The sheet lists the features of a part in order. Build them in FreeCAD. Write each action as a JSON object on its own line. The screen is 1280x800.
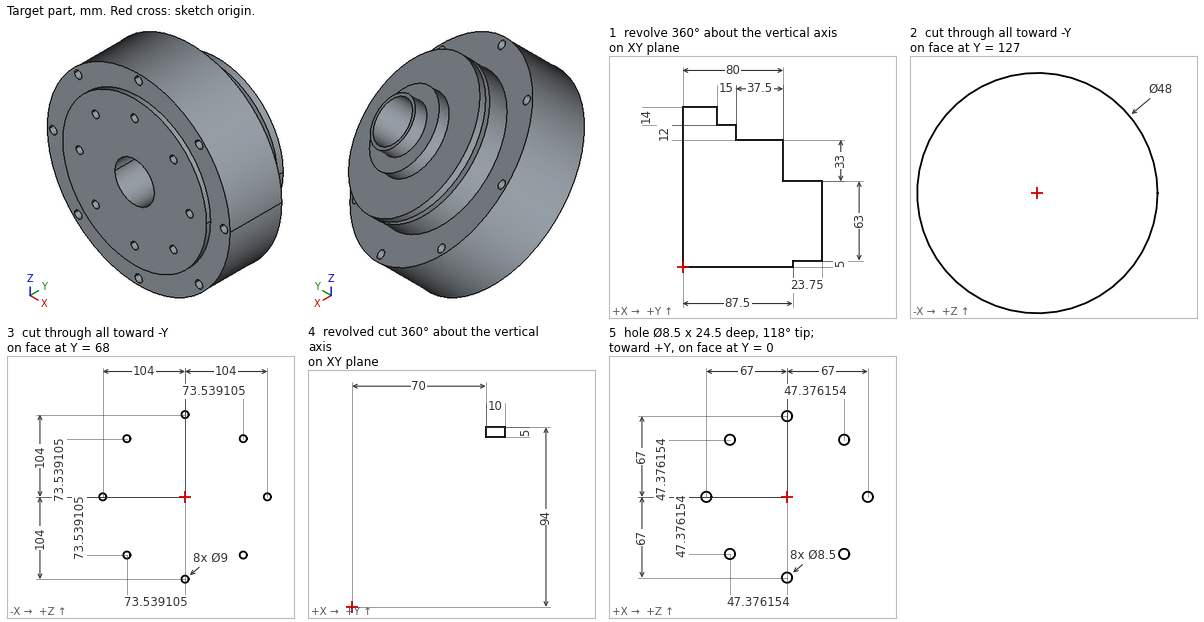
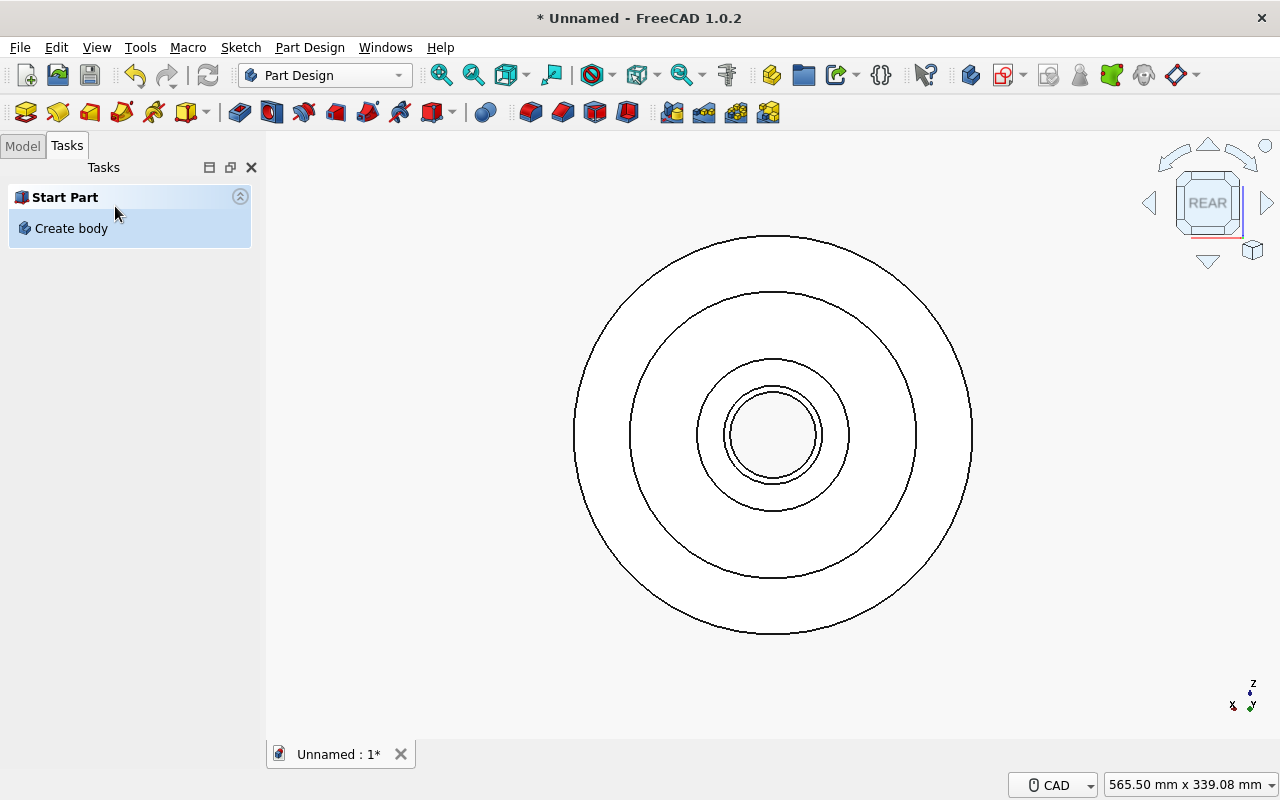
{"action": "left_click", "coordinate": [602, 434]}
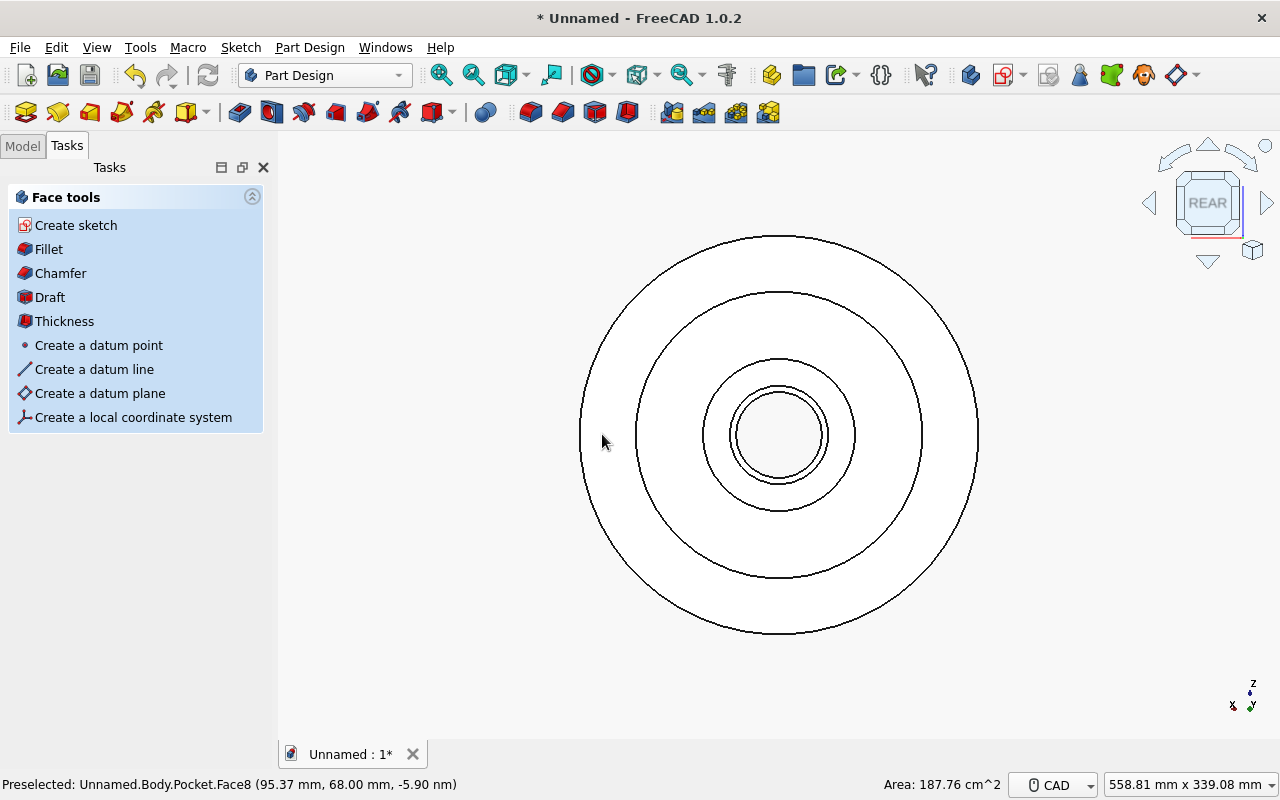
{"action": "left_click", "coordinate": [1004, 76]}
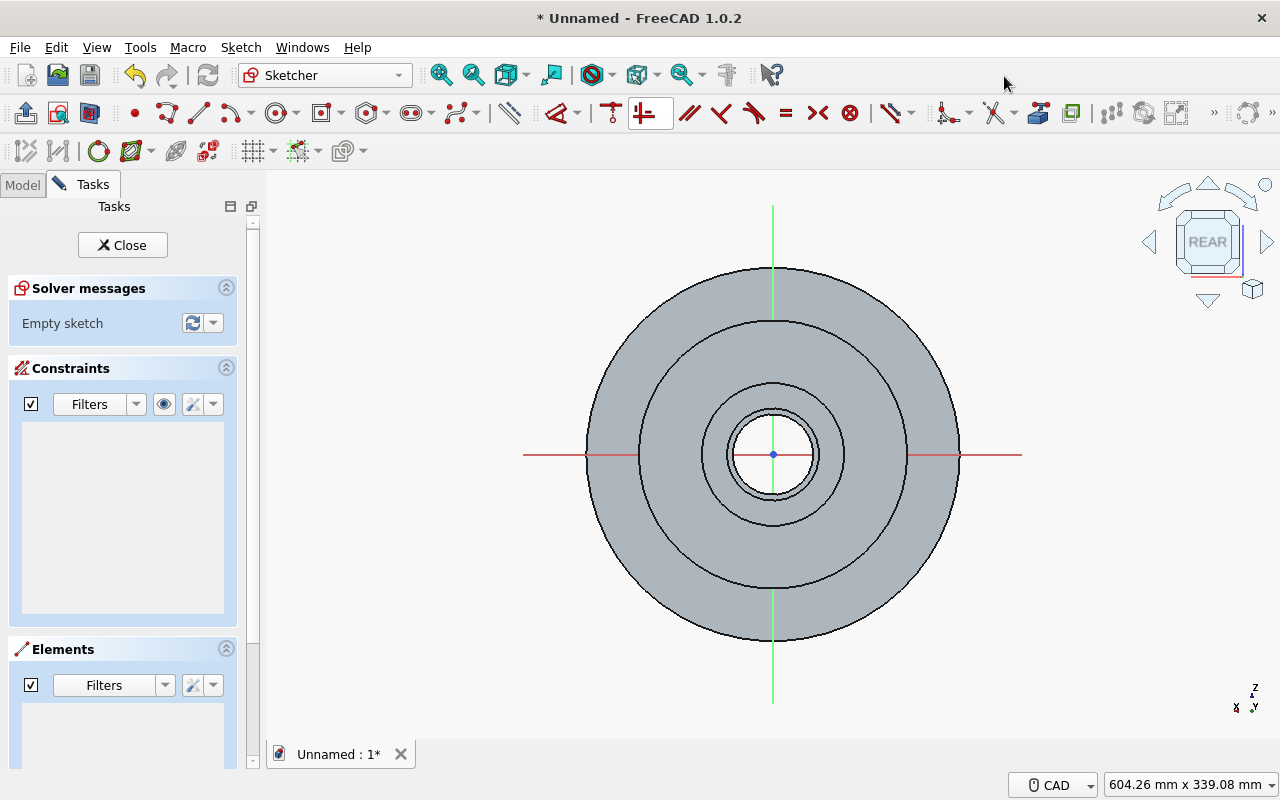
{"action": "left_click", "coordinate": [276, 114]}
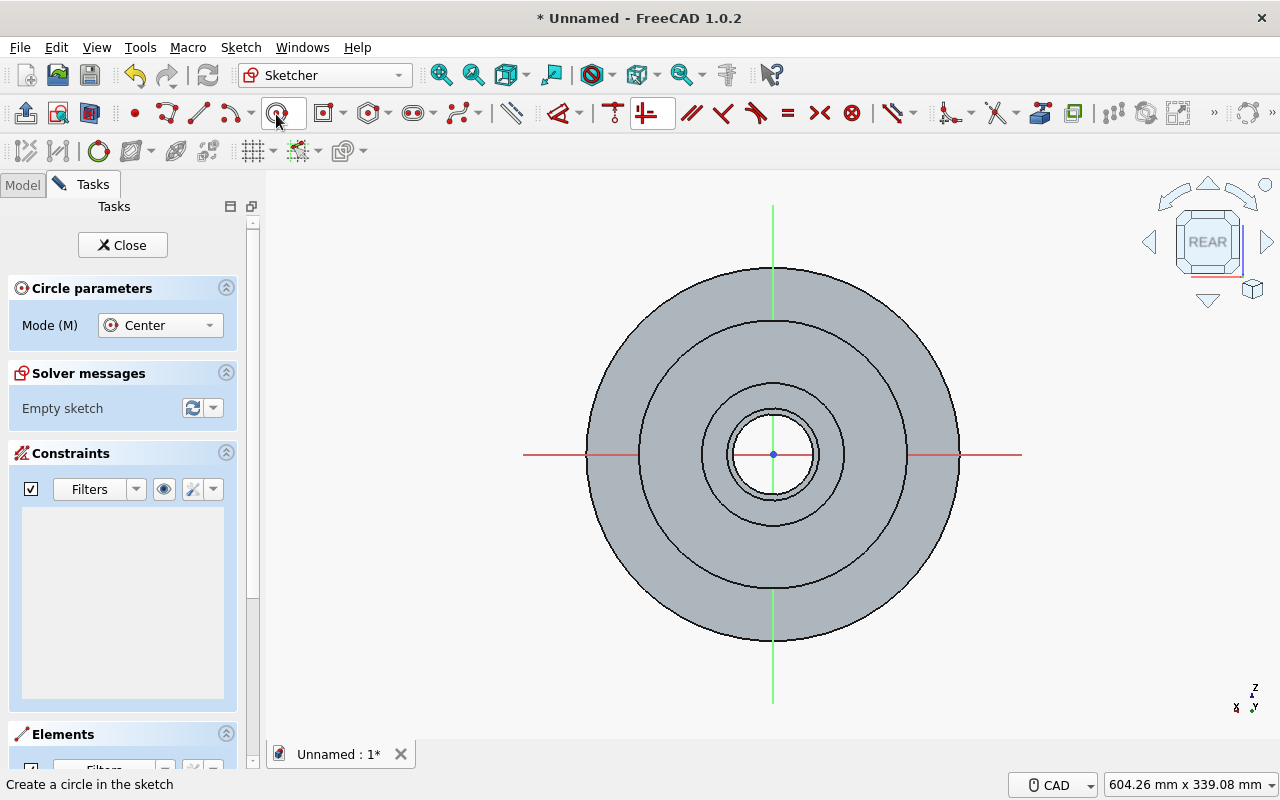
{"action": "scroll", "coordinate": [773, 629], "scroll_direction": "up", "scroll_amount": 6}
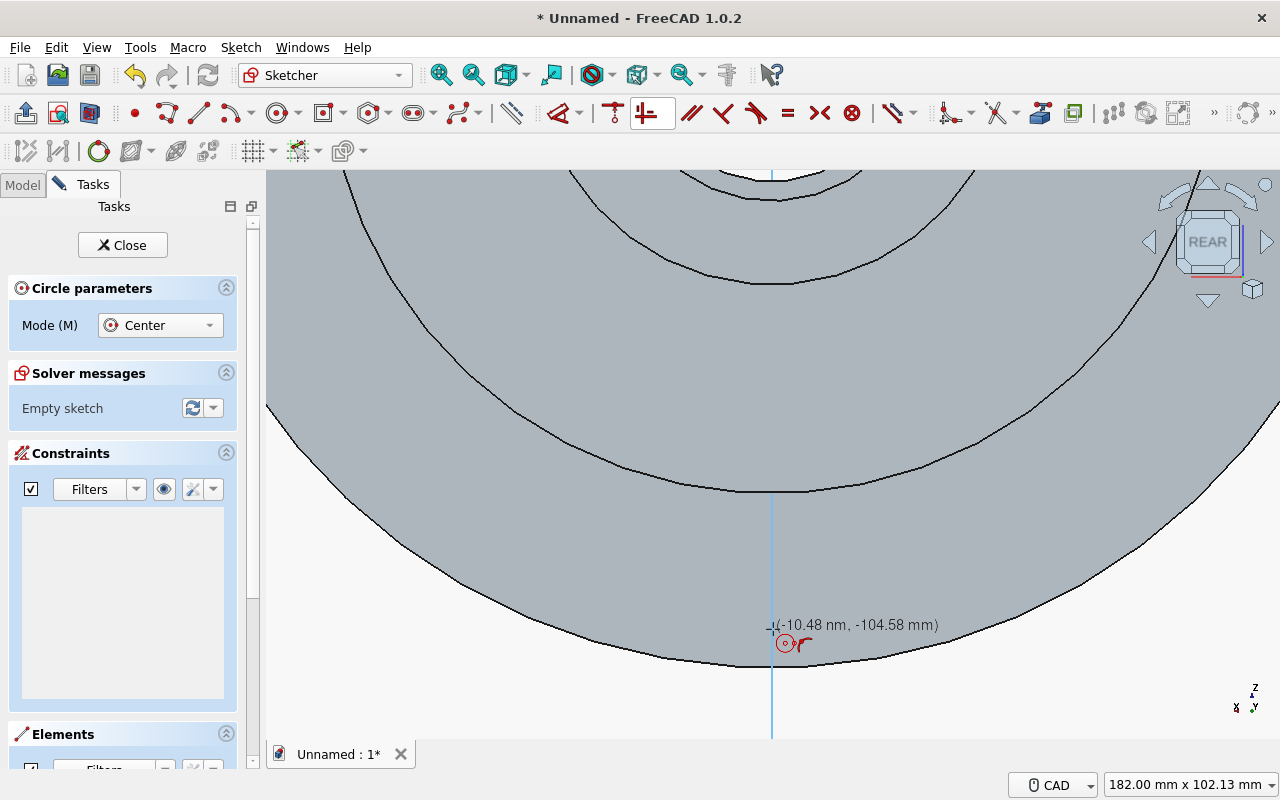
{"action": "left_click", "coordinate": [772, 627]}
{"action": "left_click", "coordinate": [790, 609]}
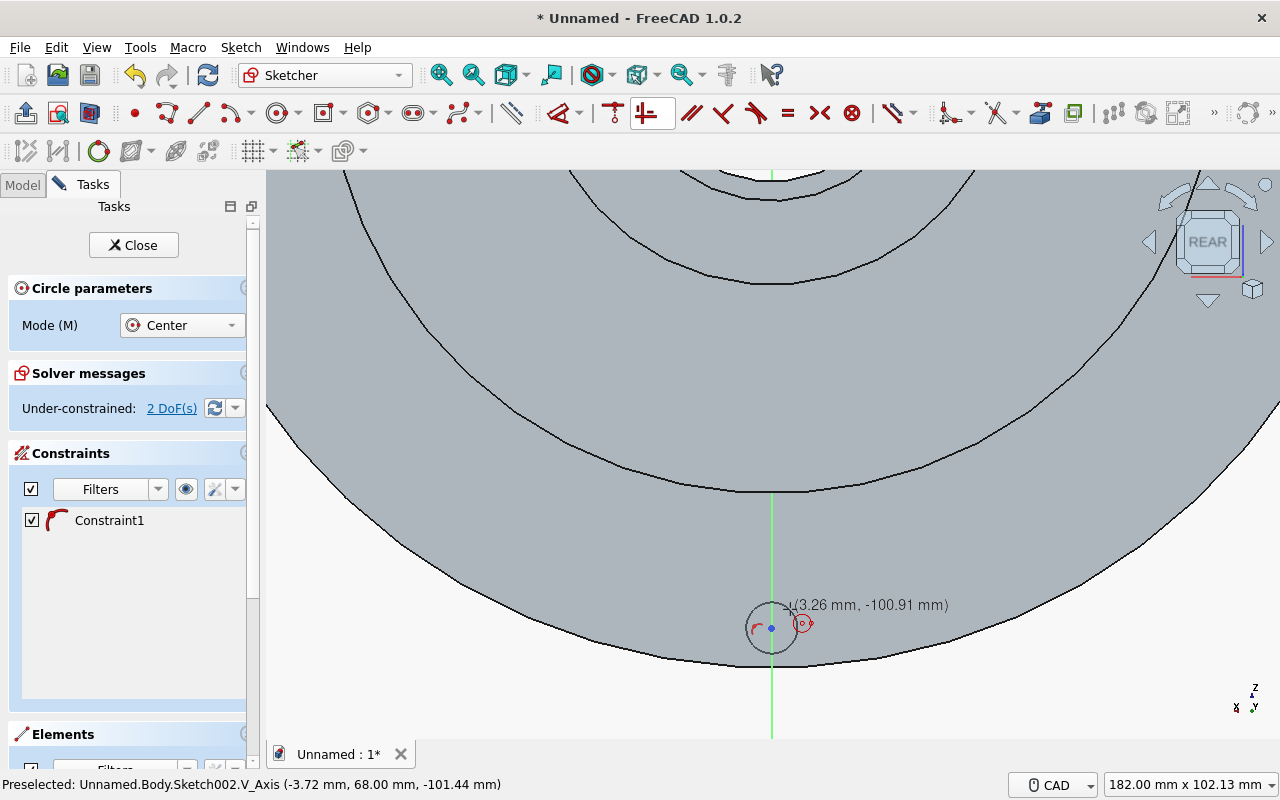
{"action": "left_click", "coordinate": [362, 457]}
{"action": "left_click", "coordinate": [380, 440]}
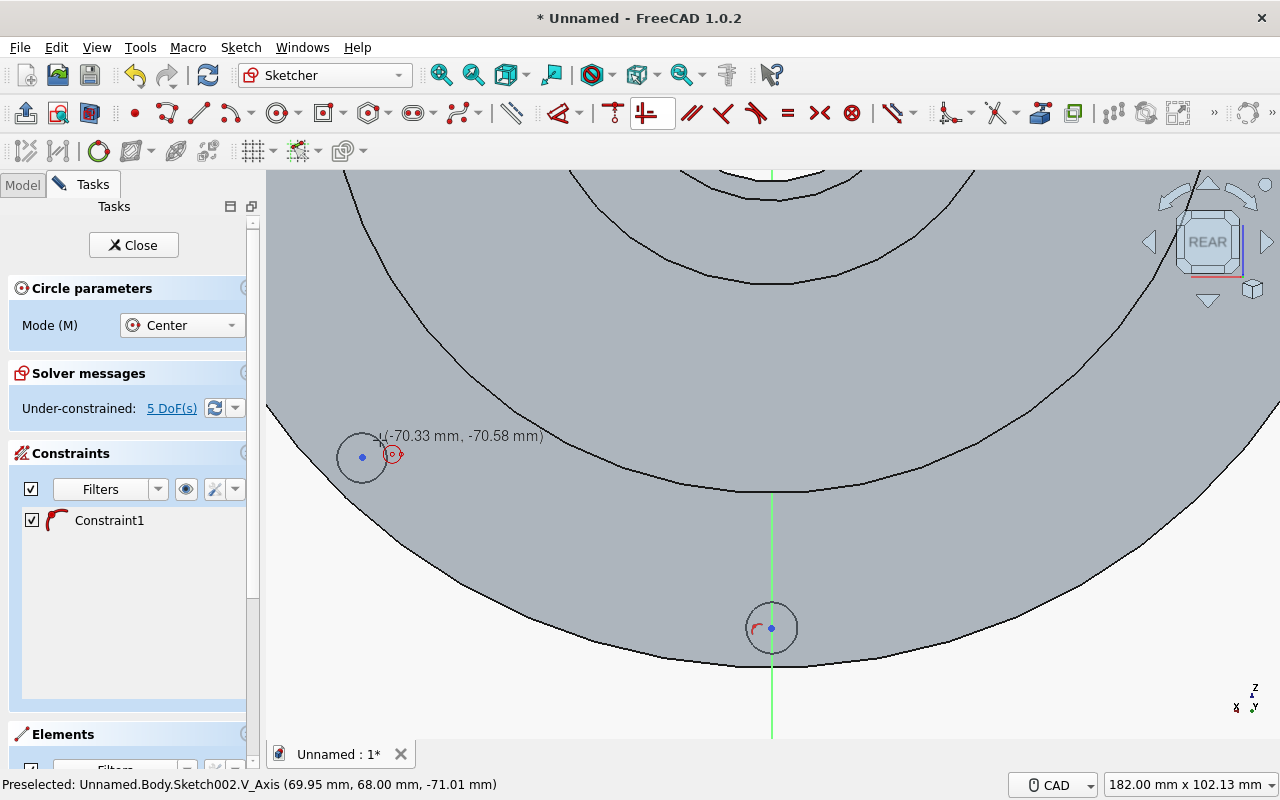
{"action": "scroll", "coordinate": [675, 630], "scroll_direction": "down", "scroll_amount": 6}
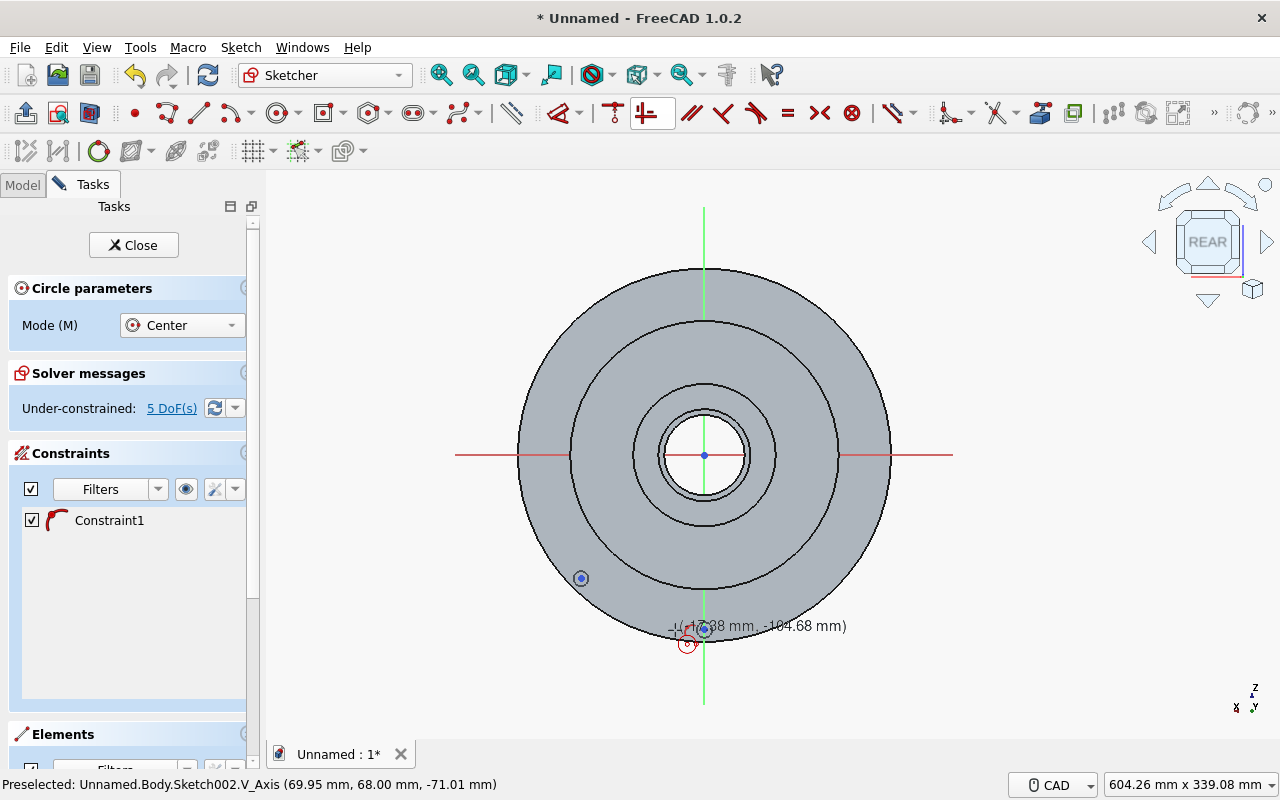
{"action": "scroll", "coordinate": [530, 455], "scroll_direction": "up", "scroll_amount": 6}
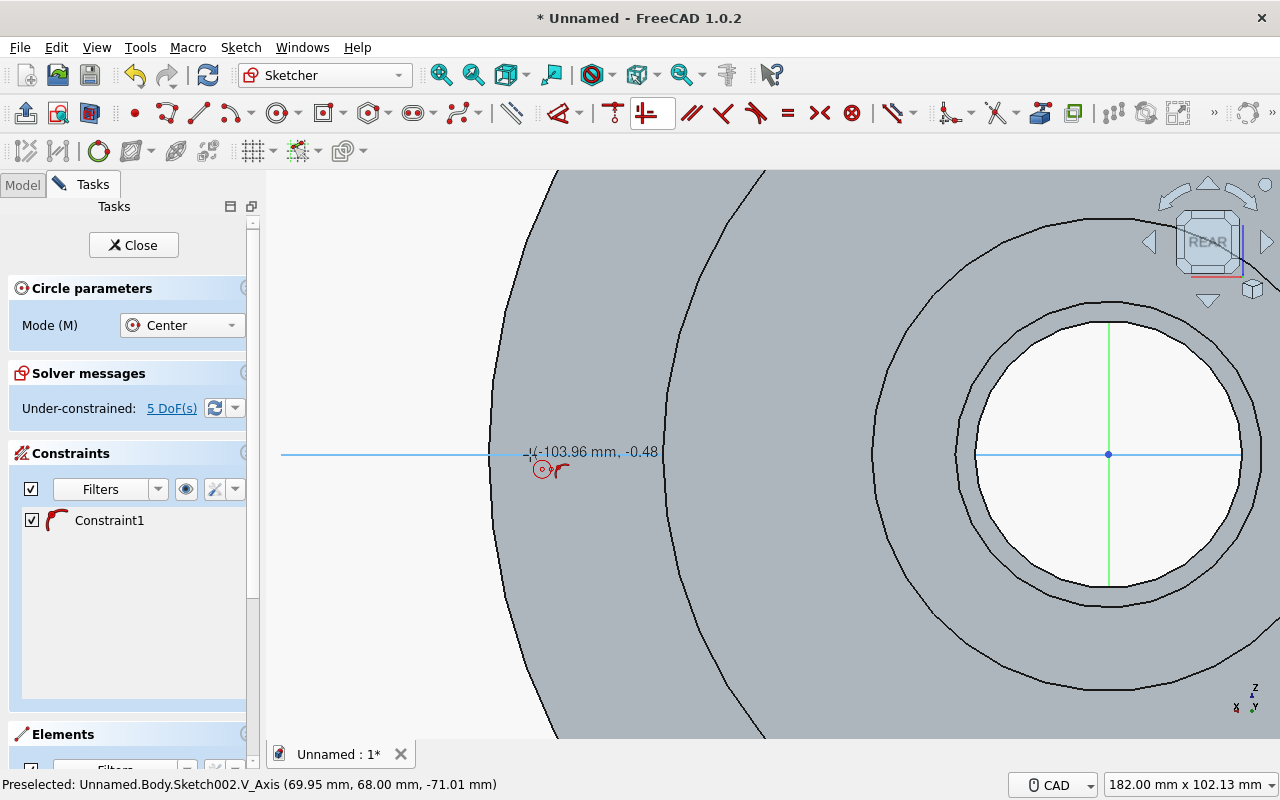
{"action": "left_click", "coordinate": [529, 455]}
{"action": "left_click", "coordinate": [547, 437]}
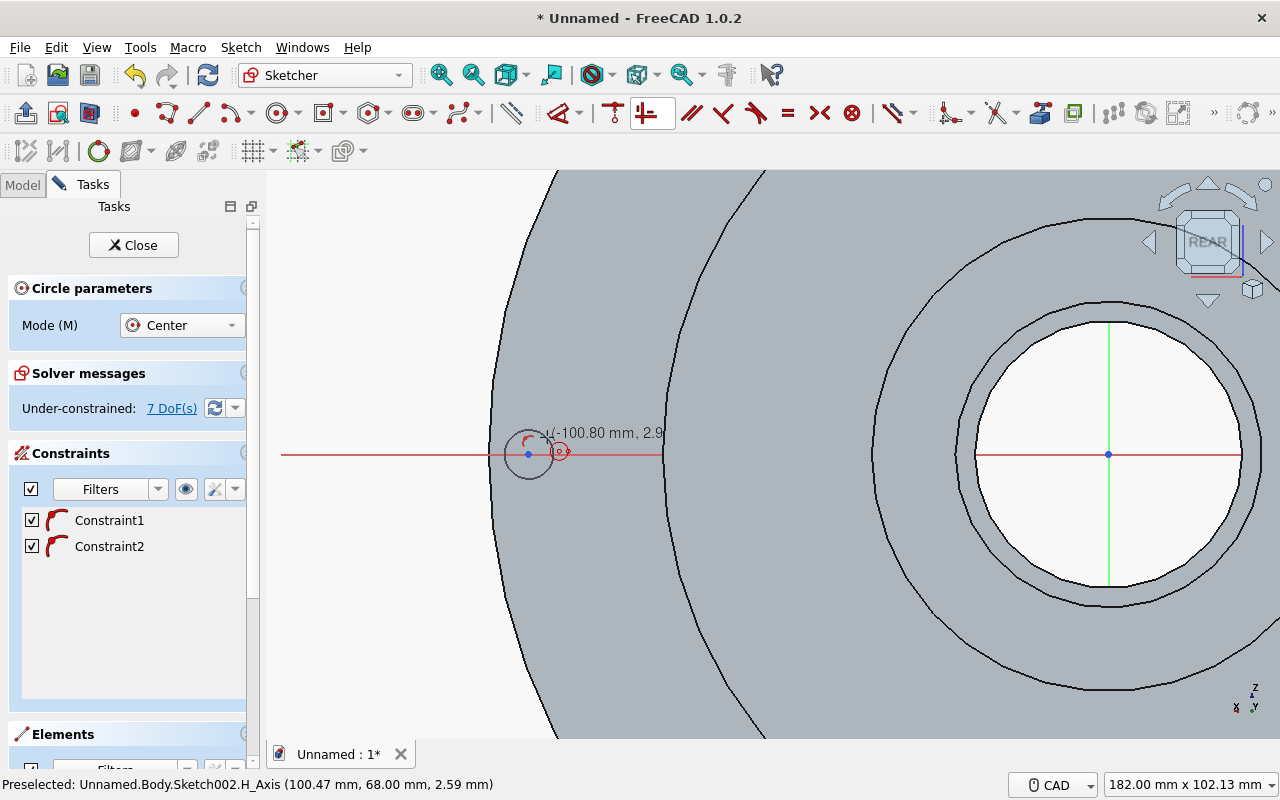
{"action": "scroll", "coordinate": [530, 454], "scroll_direction": "down", "scroll_amount": 6}